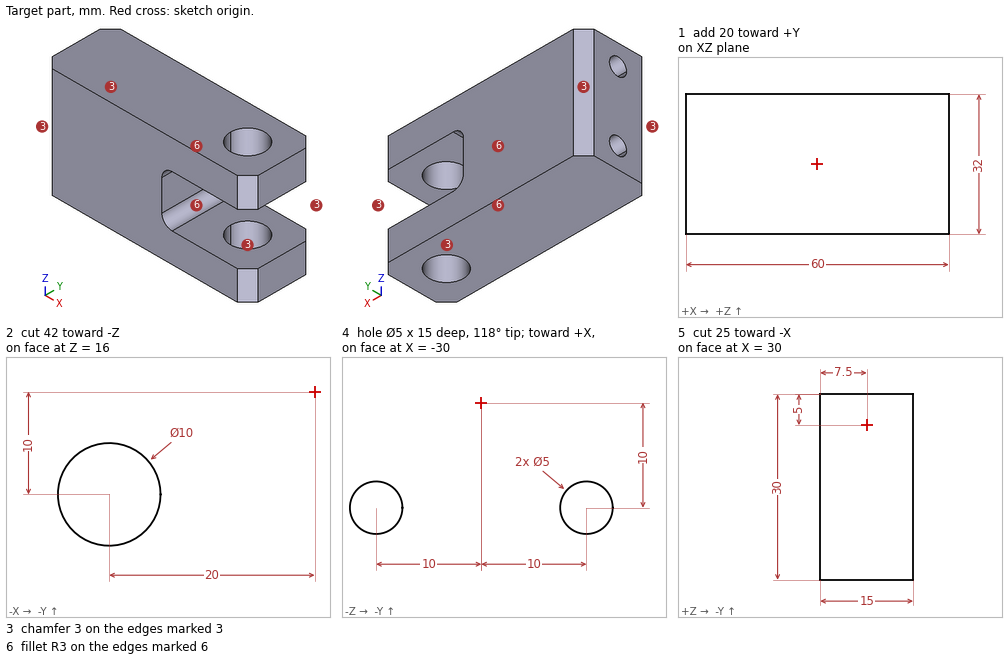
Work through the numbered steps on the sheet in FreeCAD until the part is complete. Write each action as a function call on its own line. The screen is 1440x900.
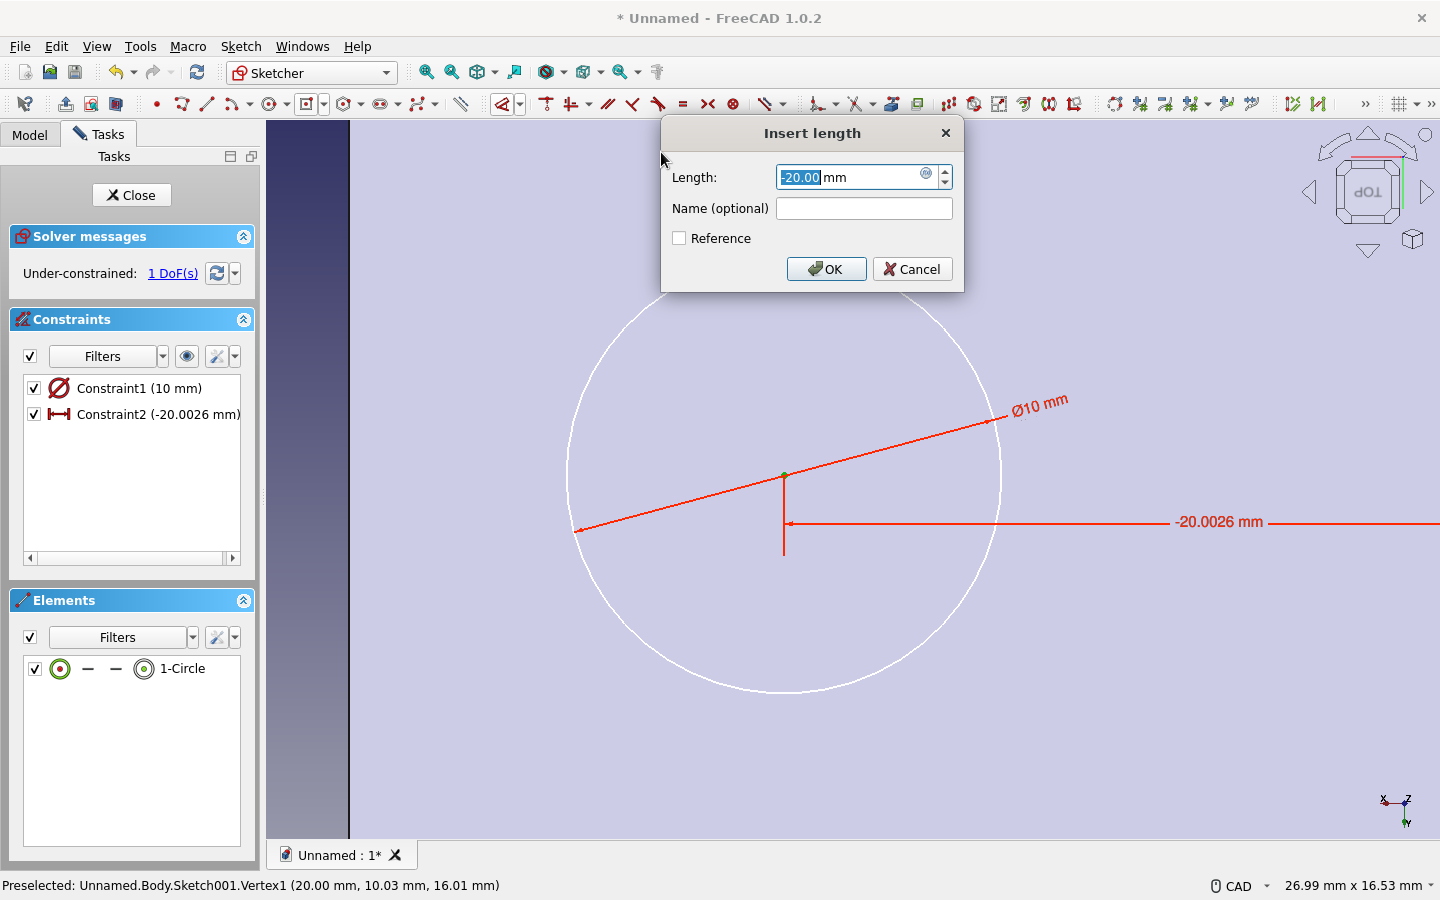
text(-20)
key(Return)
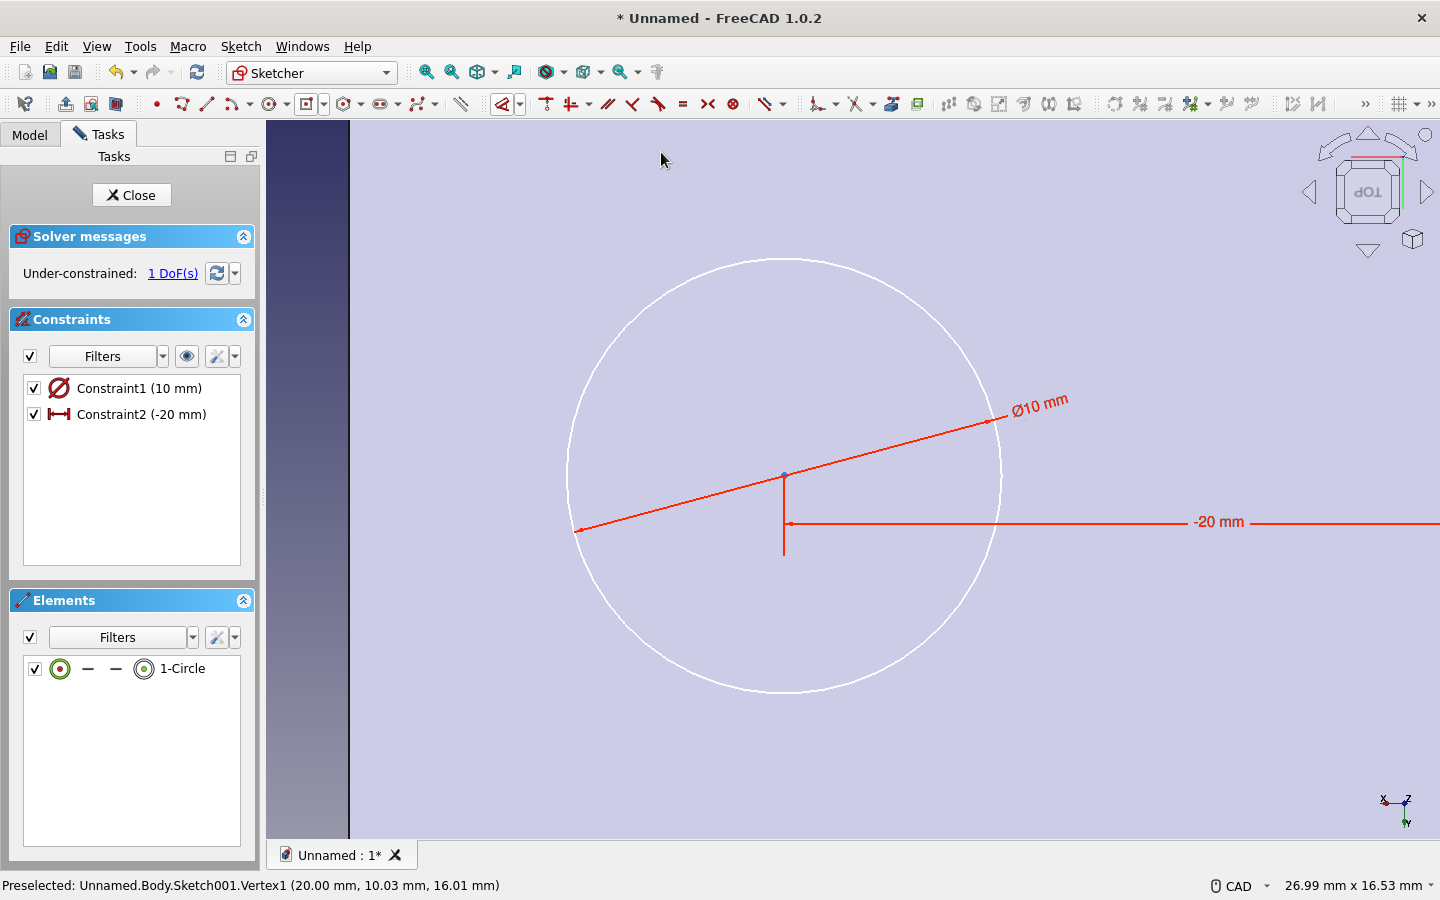
click(784, 476)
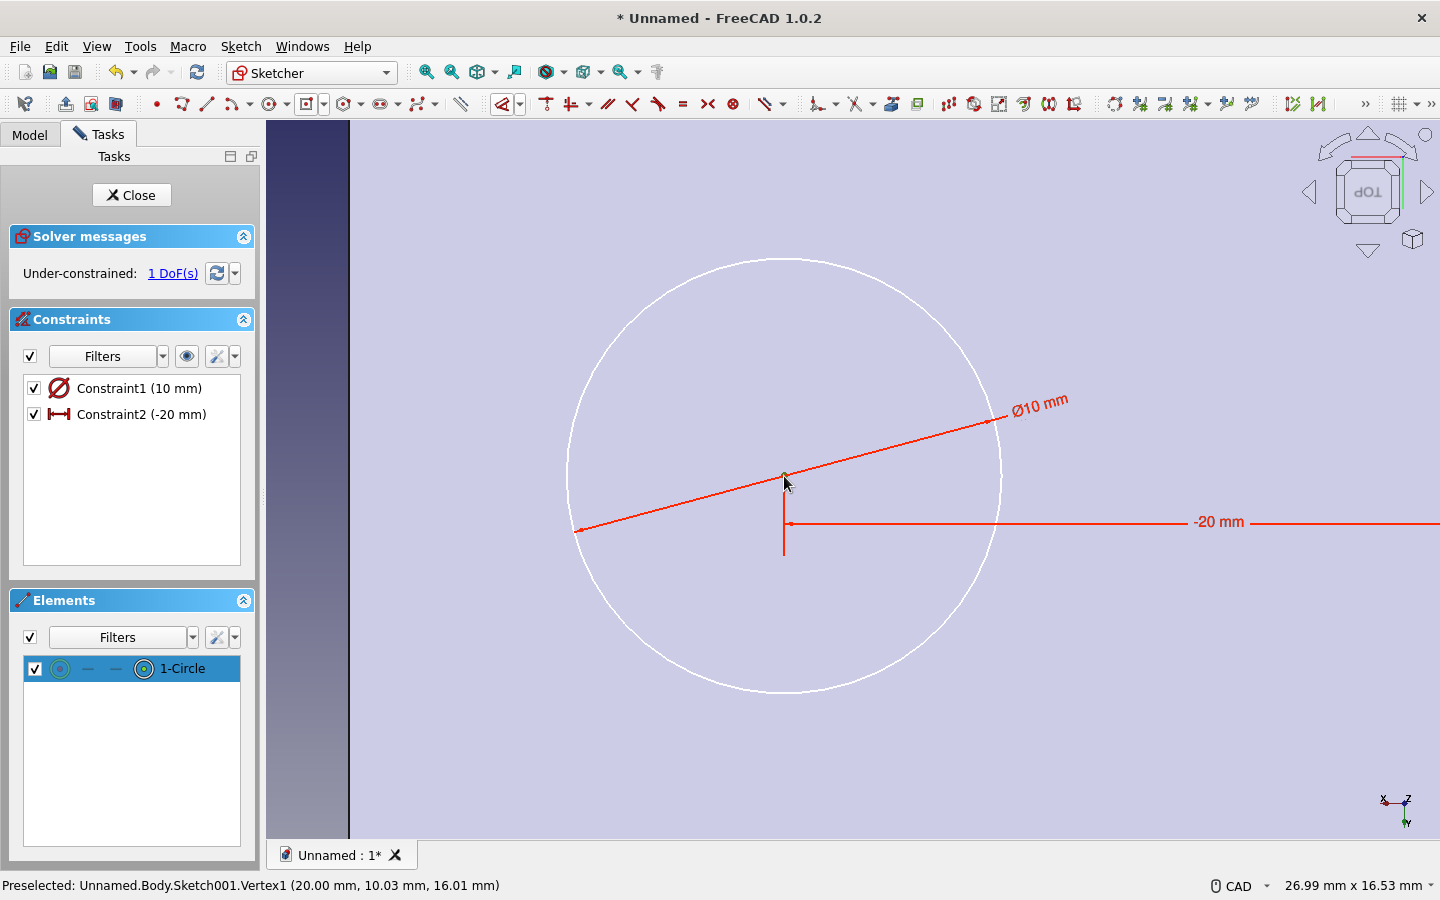
key(i)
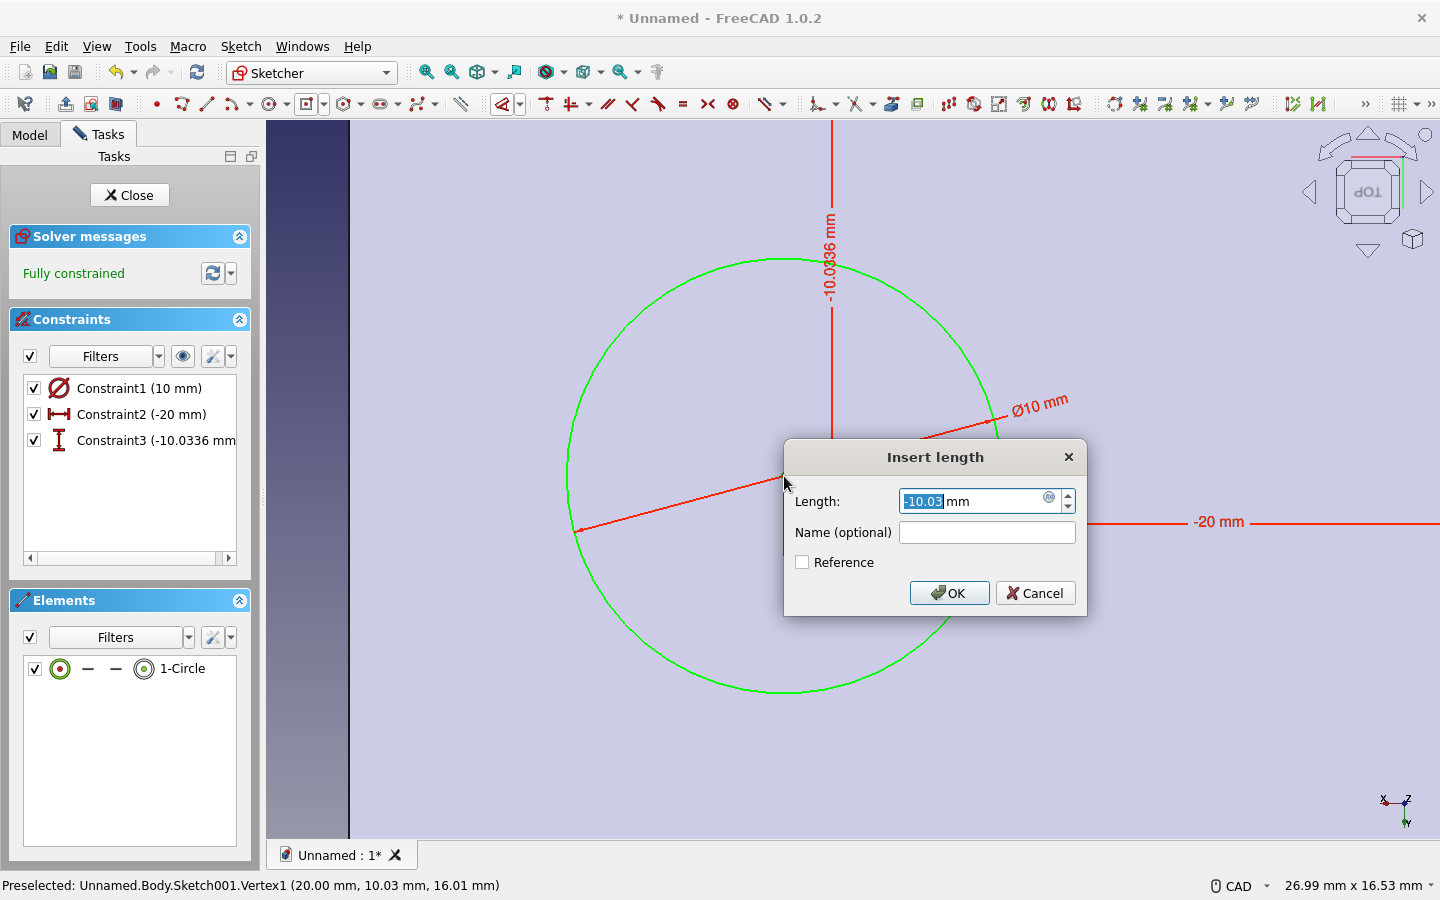
text(-10)
key(Return)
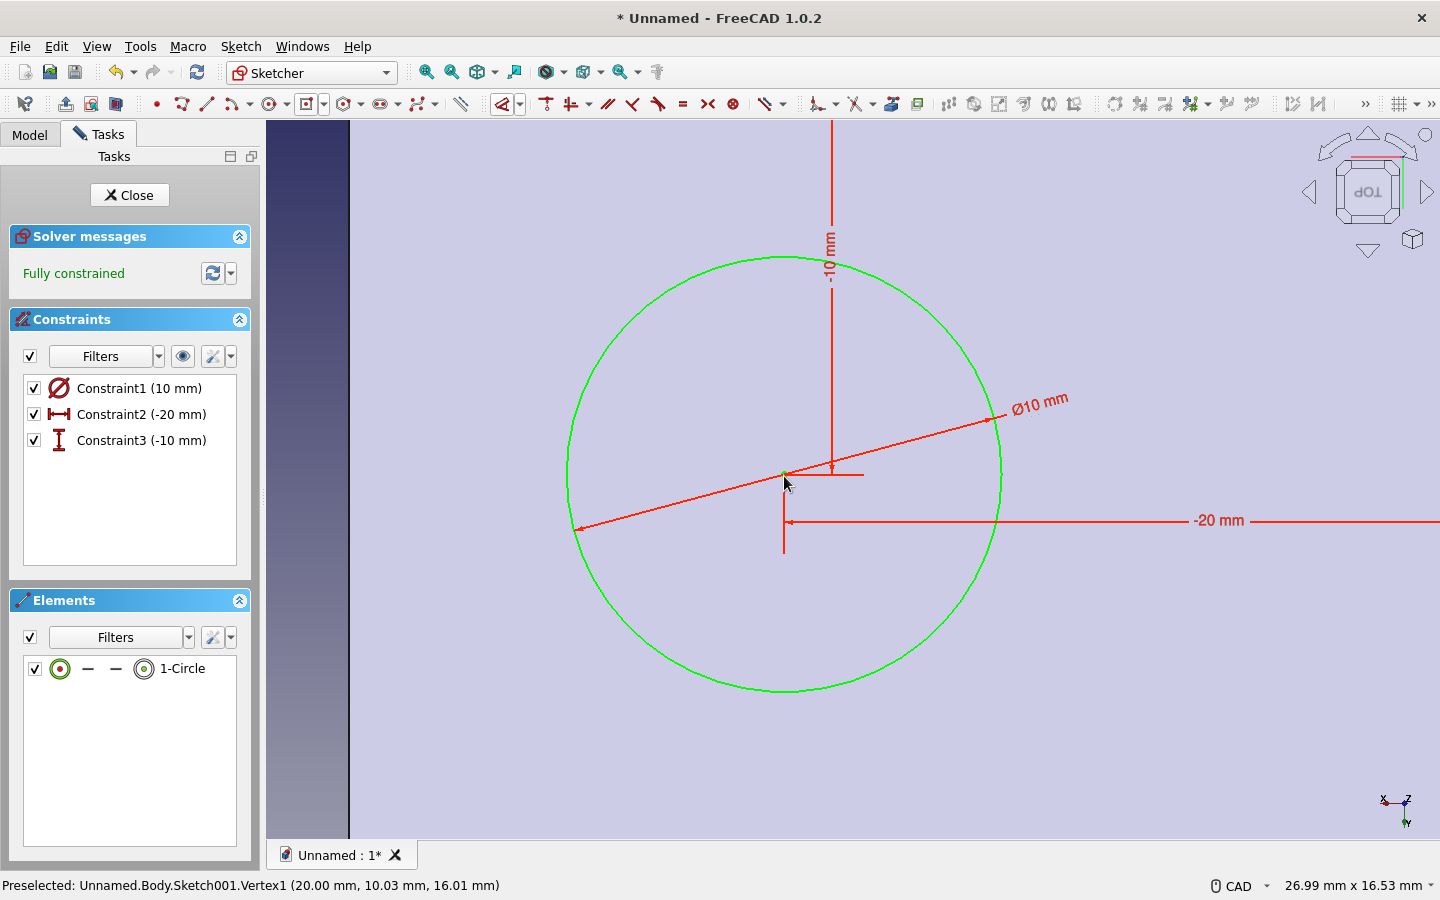
click(130, 195)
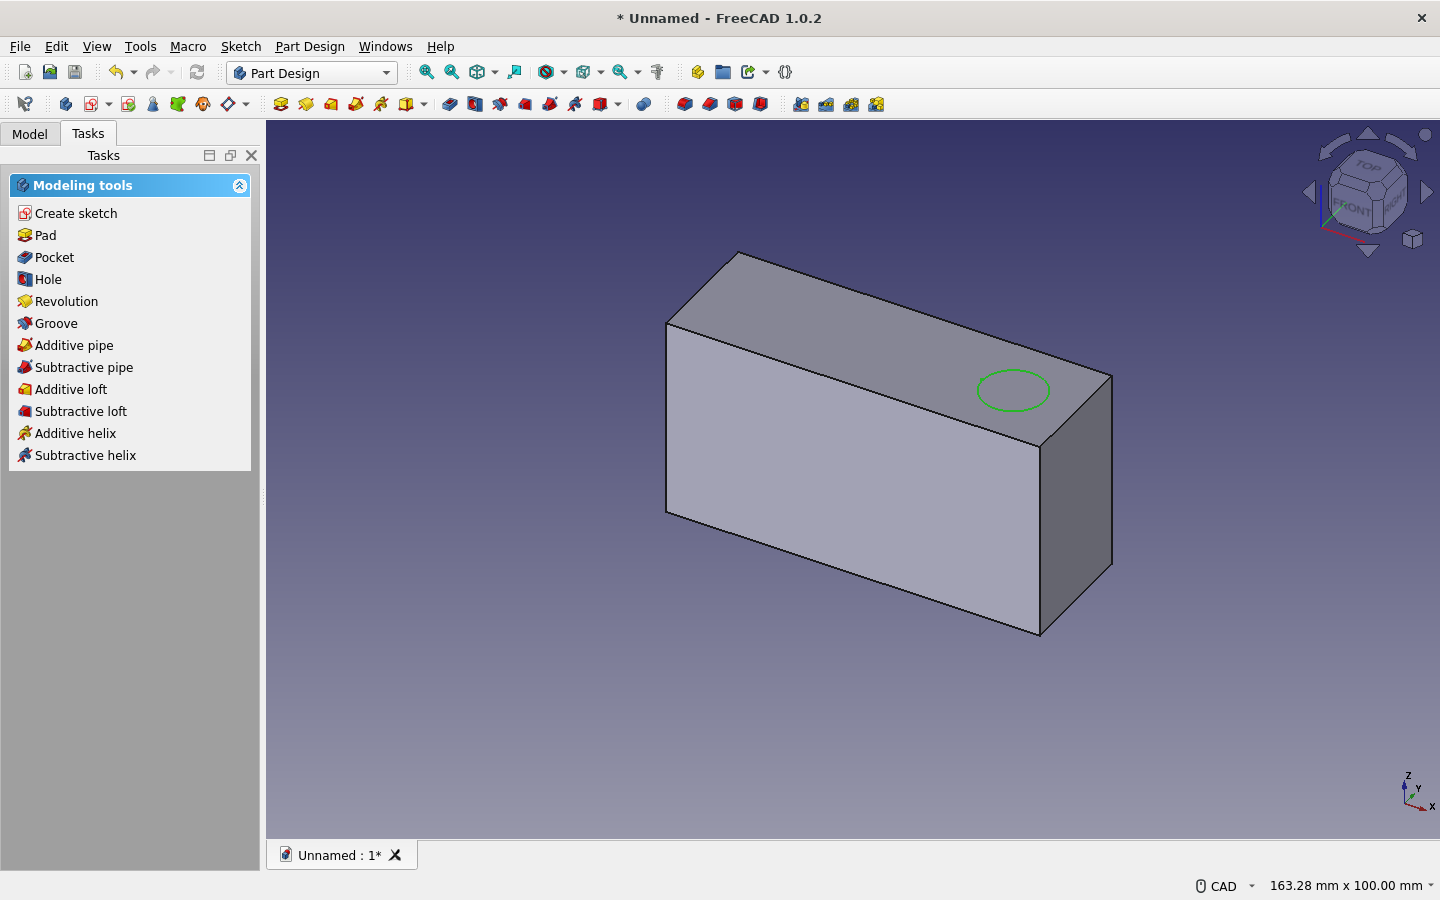
click(450, 104)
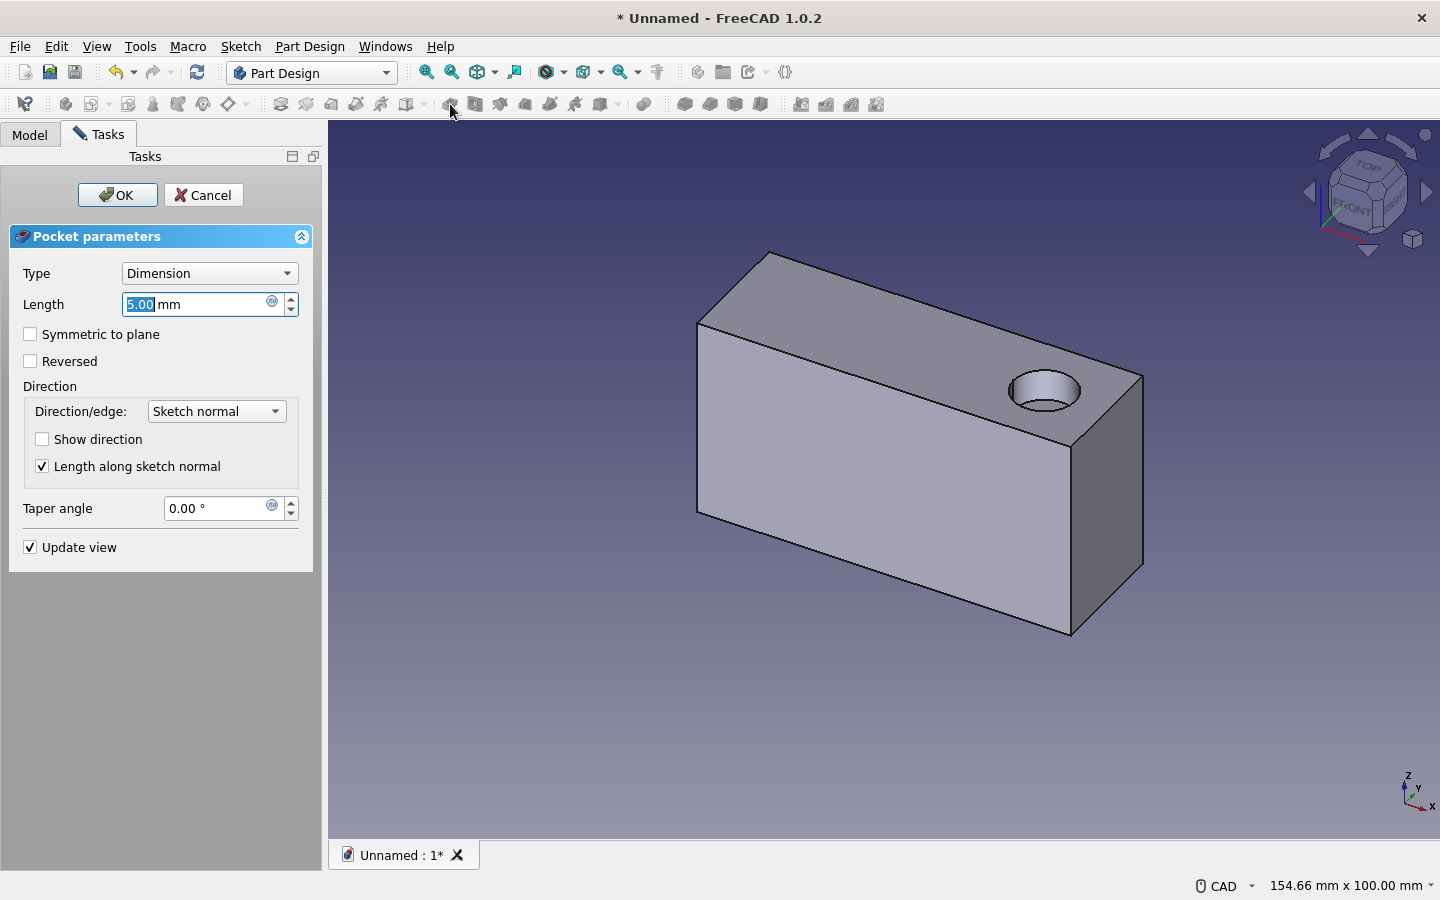
text(42)
key(Tab)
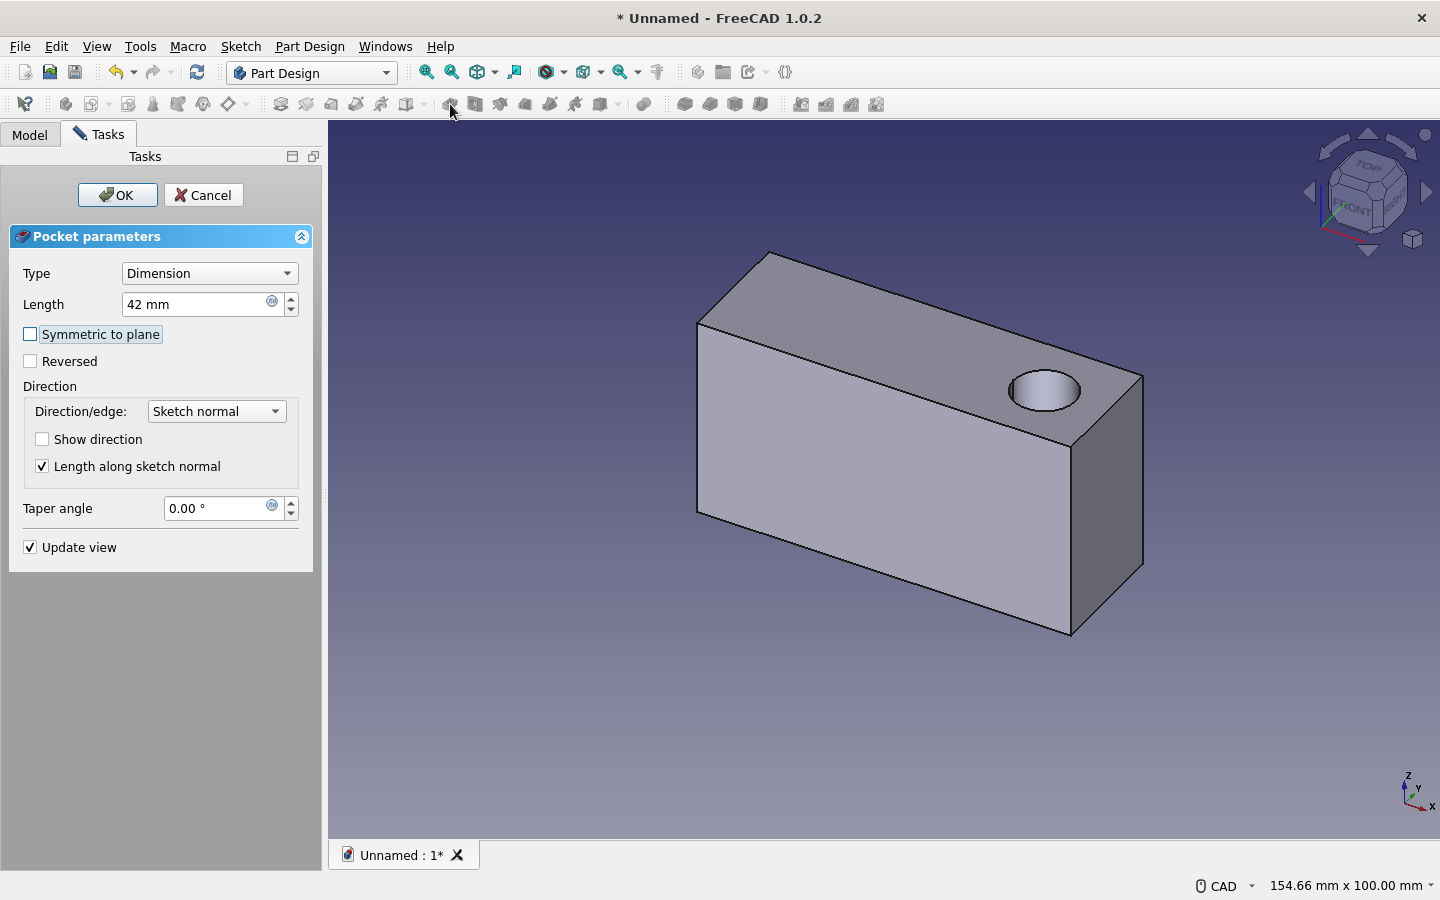
click(118, 195)